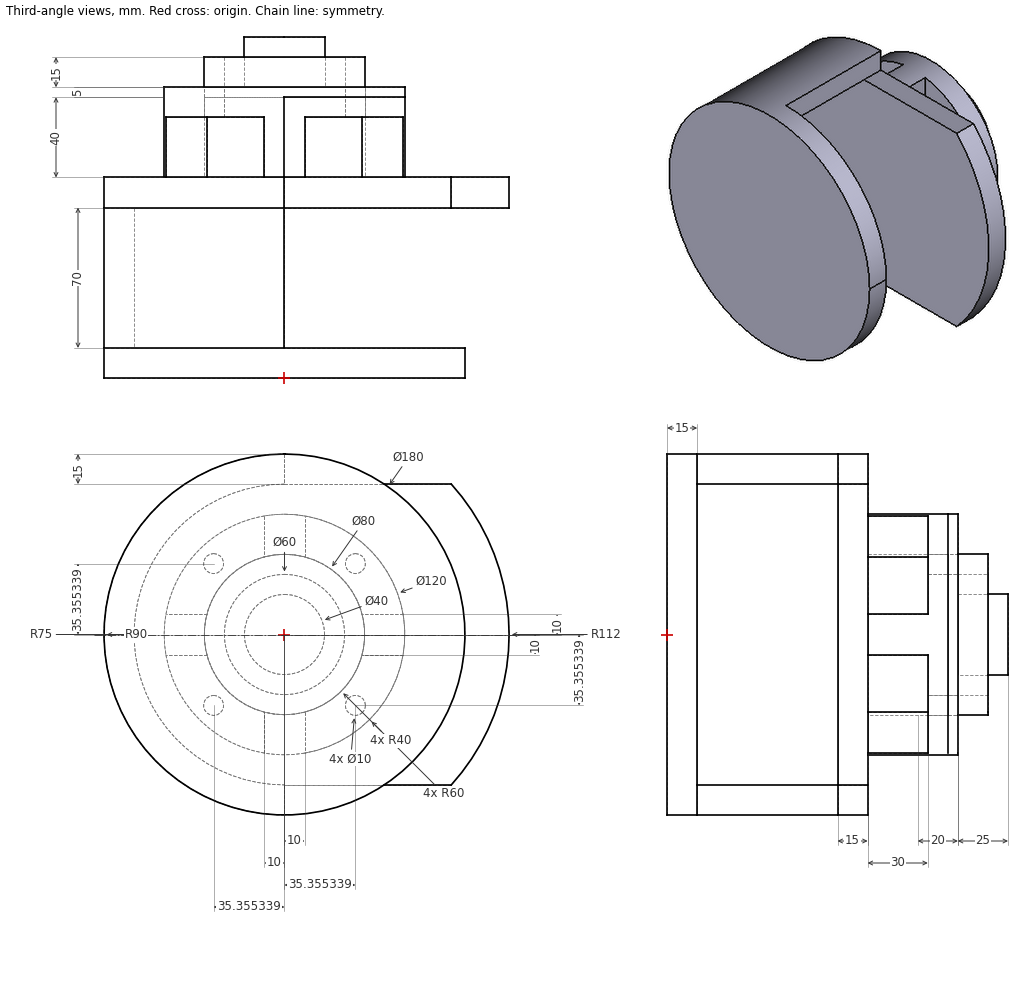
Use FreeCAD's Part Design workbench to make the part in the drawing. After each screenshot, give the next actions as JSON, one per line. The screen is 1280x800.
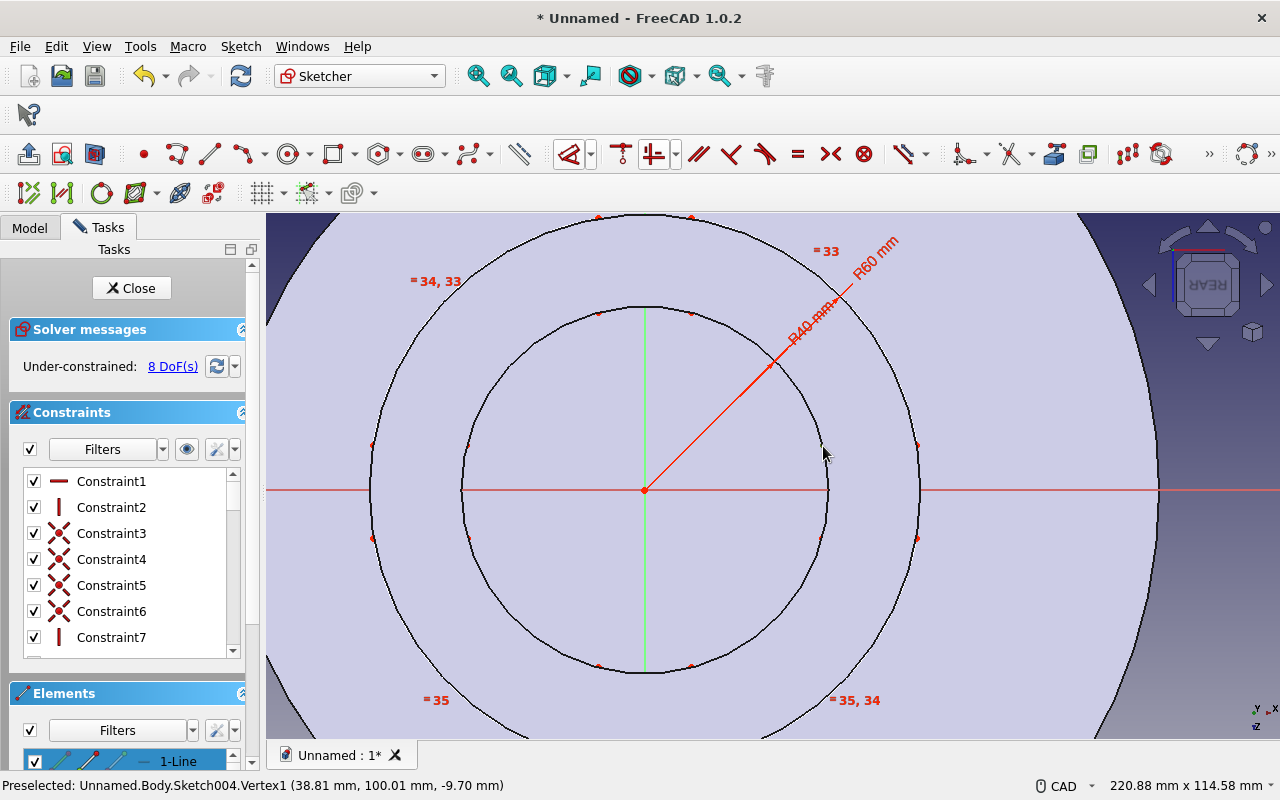
{"action": "left_click", "coordinate": [590, 154]}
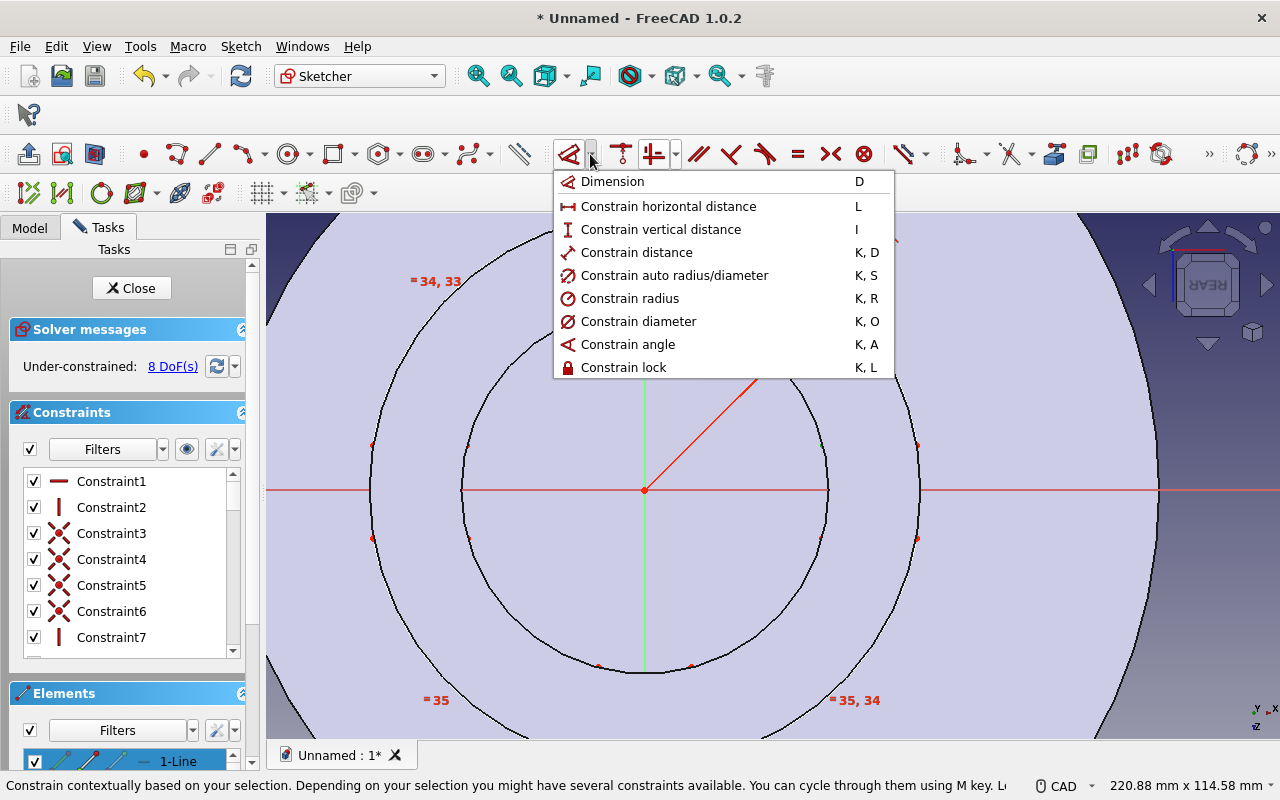
{"action": "left_click", "coordinate": [724, 230]}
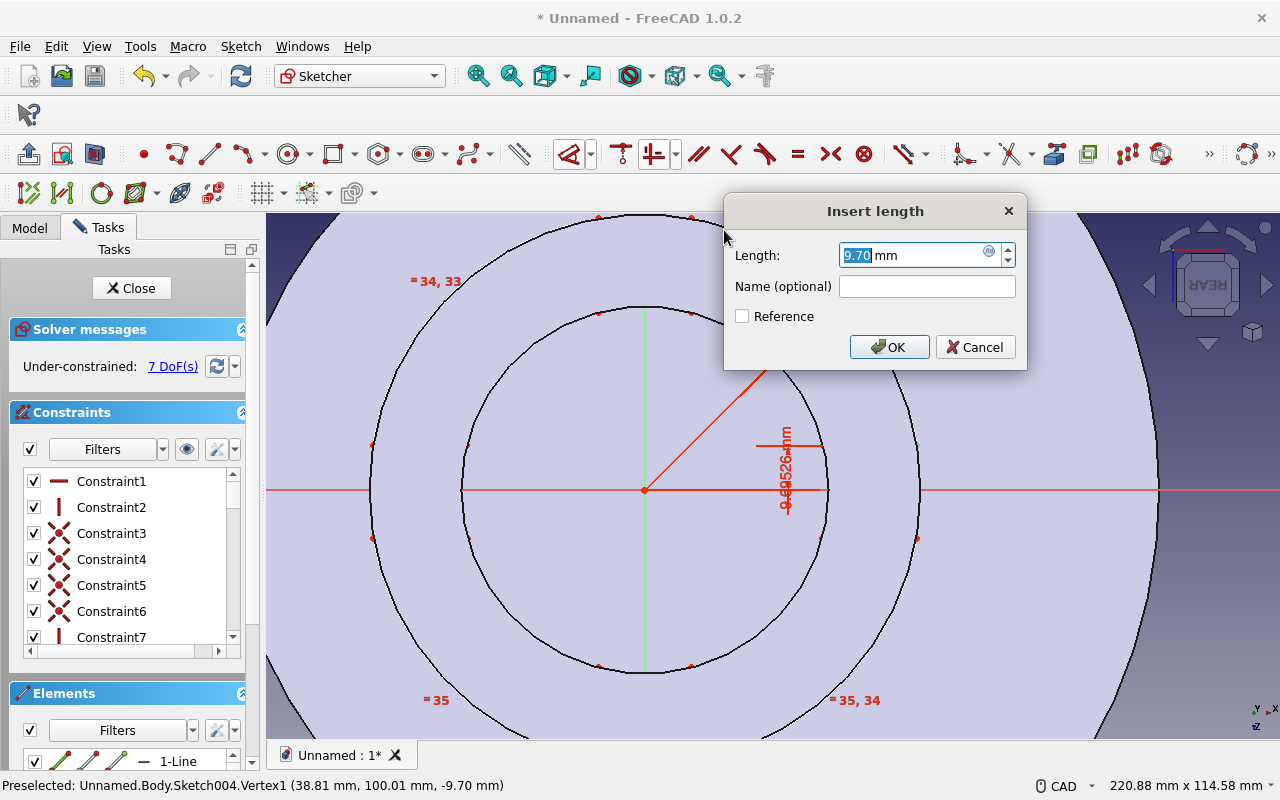
{"action": "type", "text": "10"}
{"action": "key", "text": "Return"}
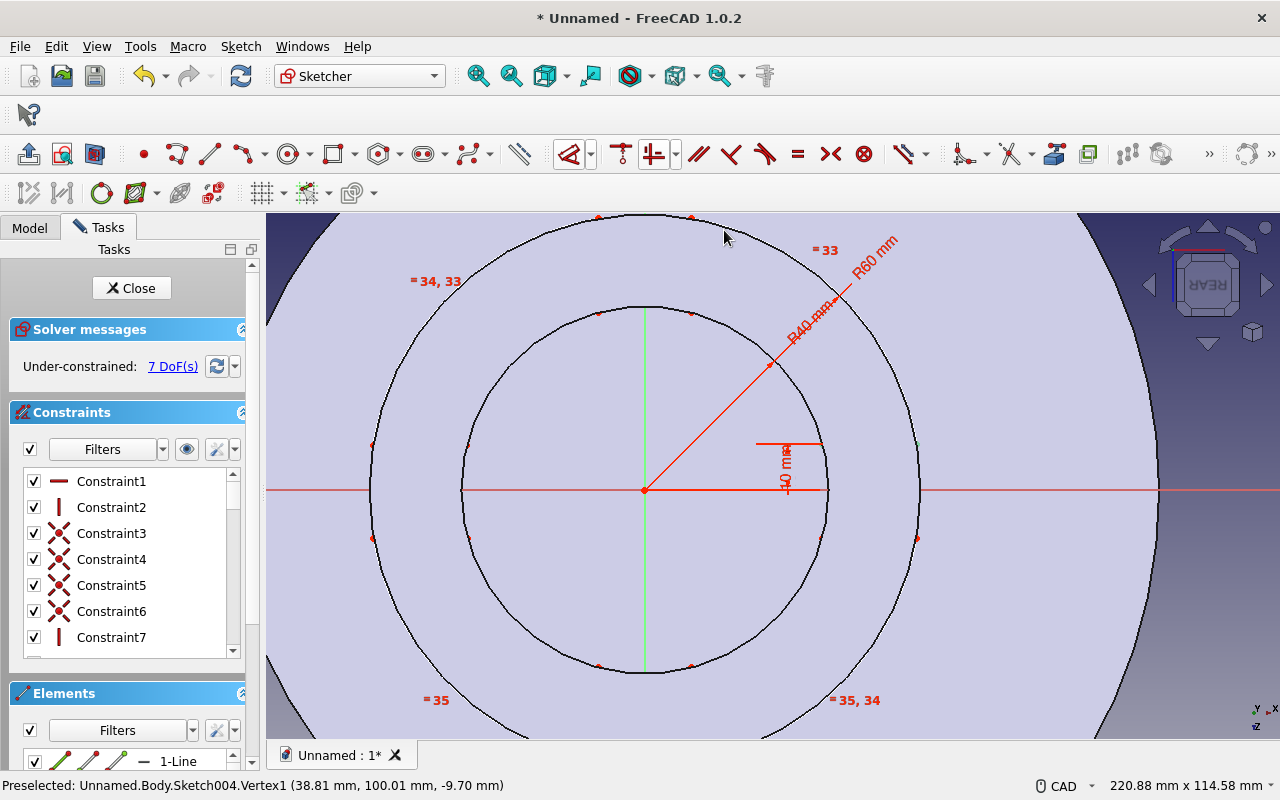
{"action": "scroll", "coordinate": [826, 447], "scroll_direction": "down", "scroll_amount": 2}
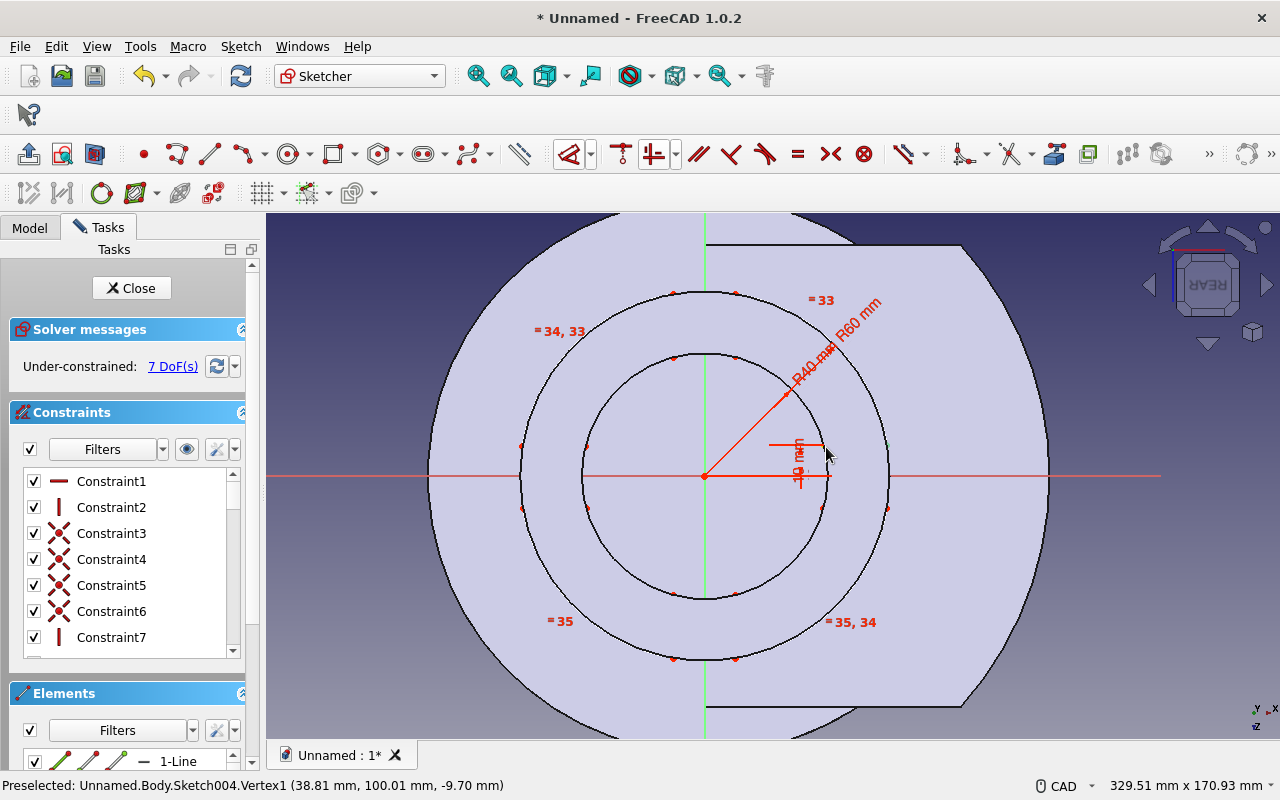
{"action": "scroll", "coordinate": [736, 294], "scroll_direction": "up", "scroll_amount": 2}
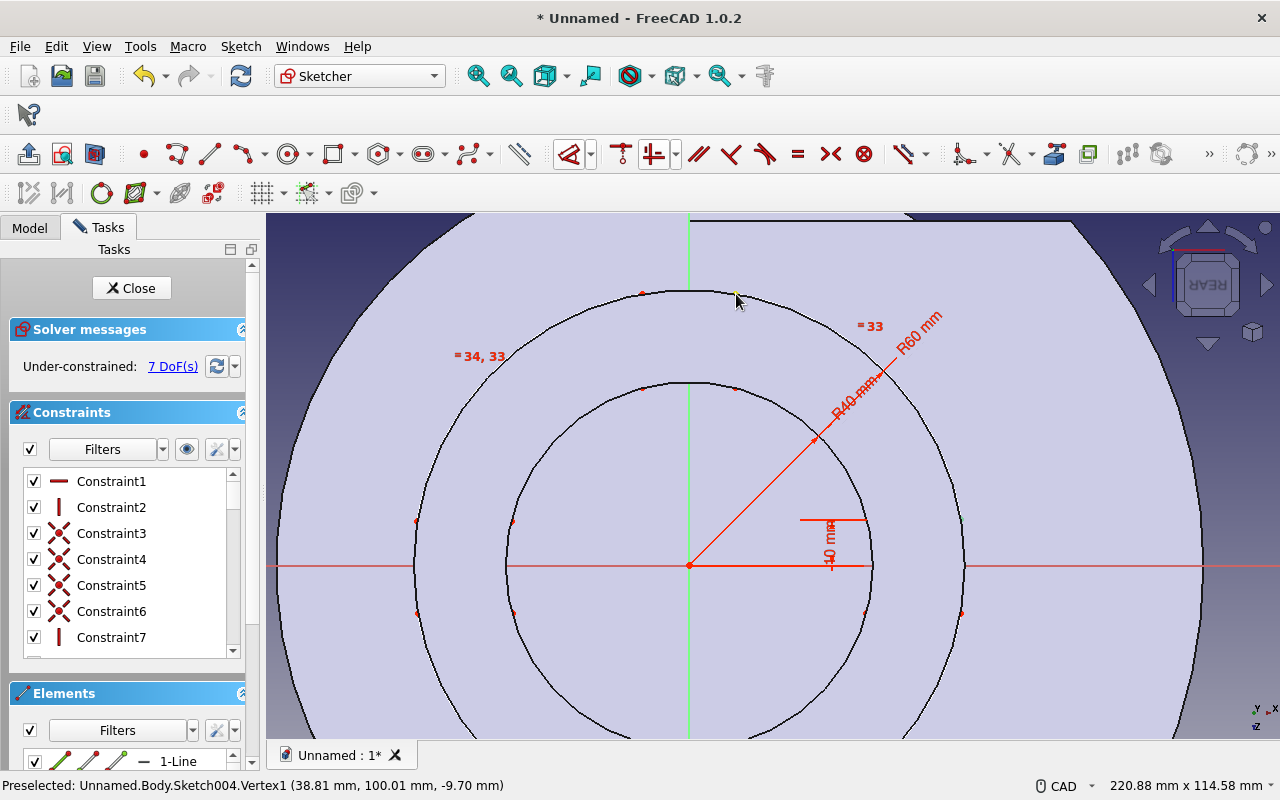
{"action": "left_click", "coordinate": [735, 294]}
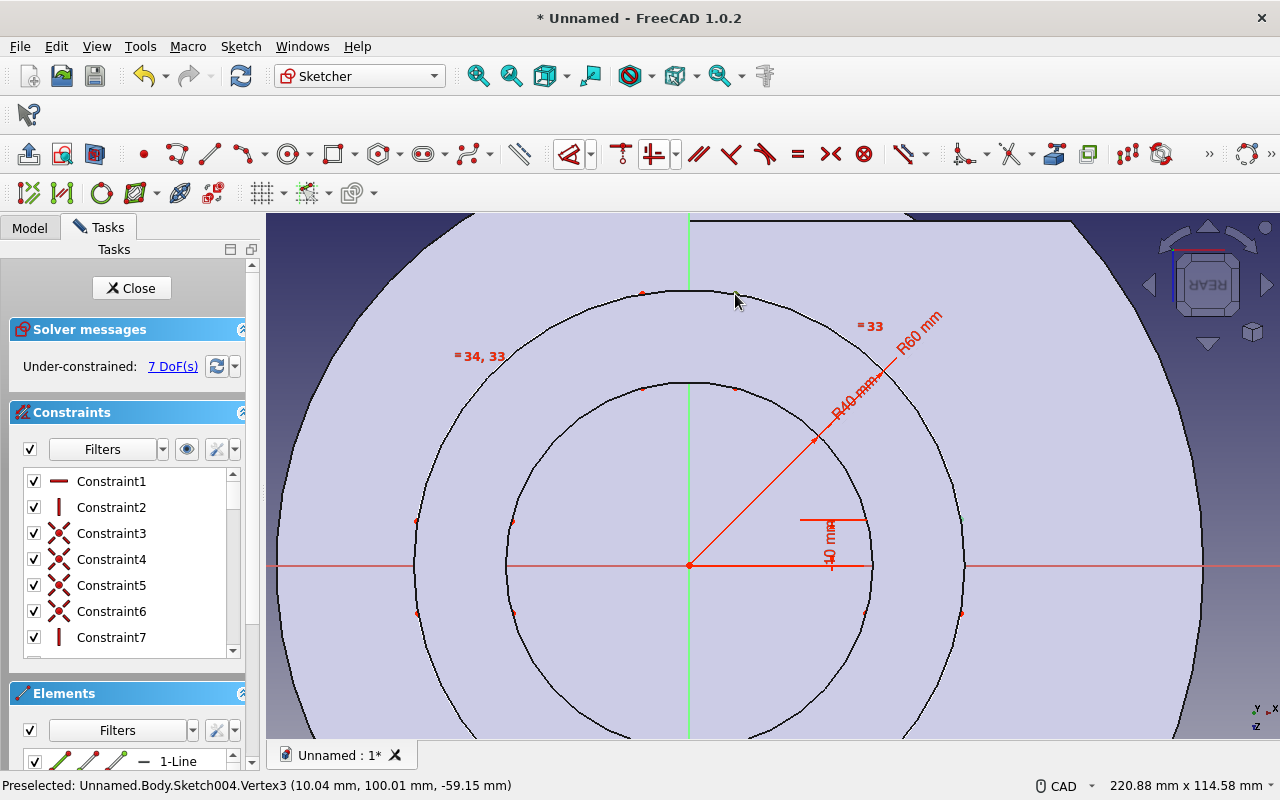
{"action": "left_click", "coordinate": [590, 154]}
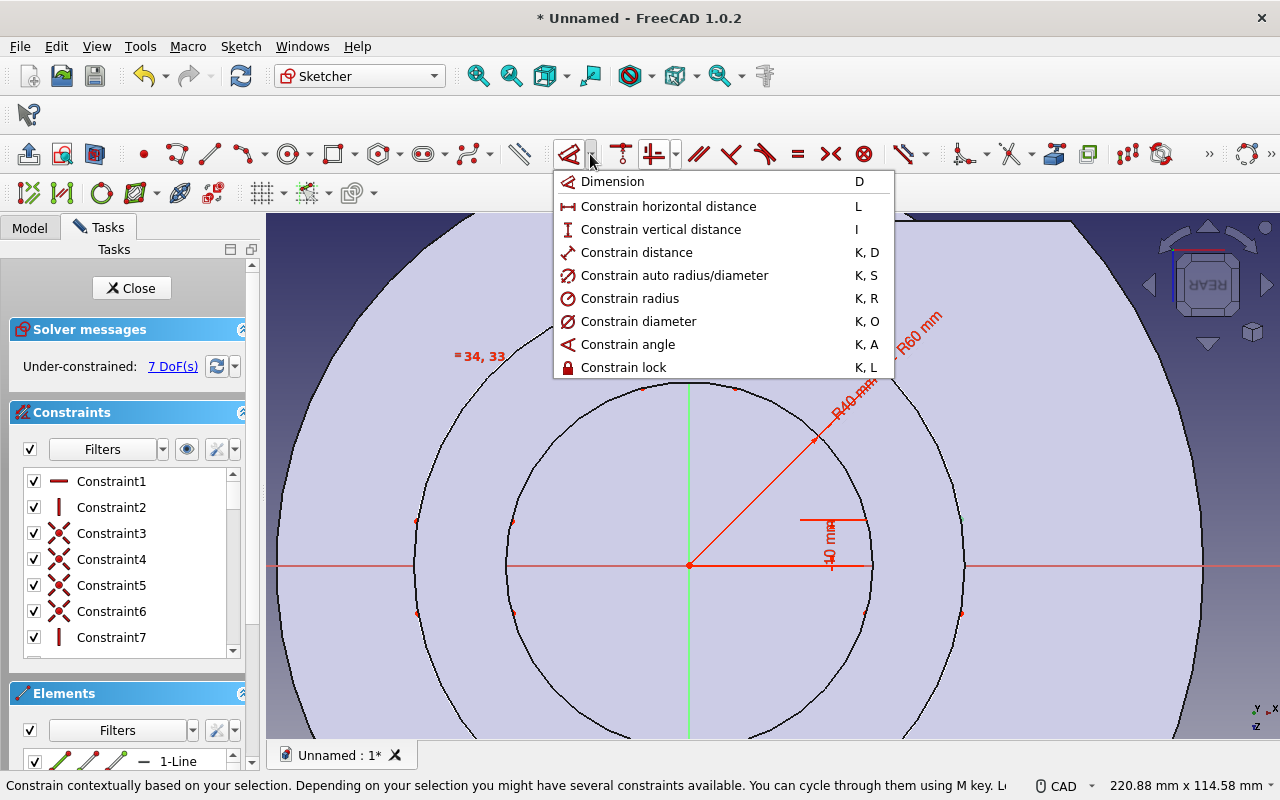
{"action": "left_click", "coordinate": [724, 206]}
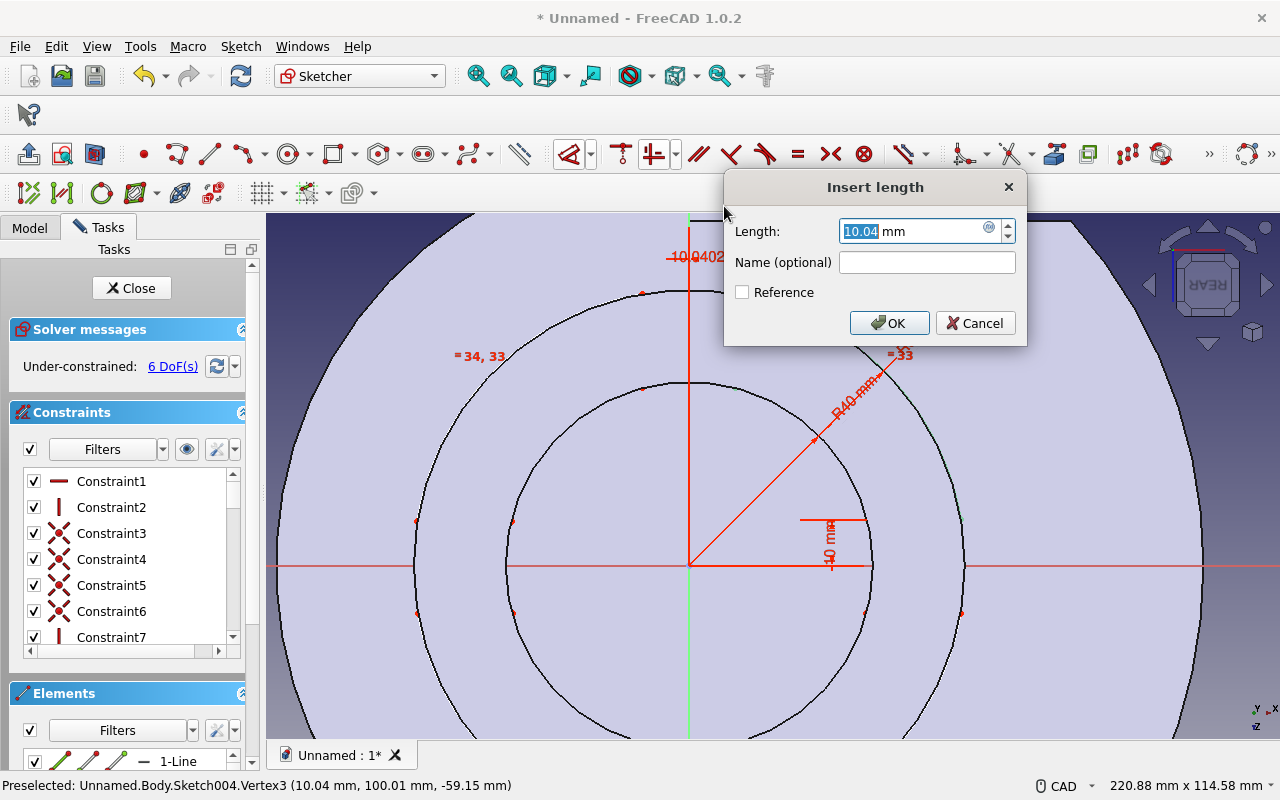
{"action": "type", "text": "10"}
{"action": "key", "text": "Return"}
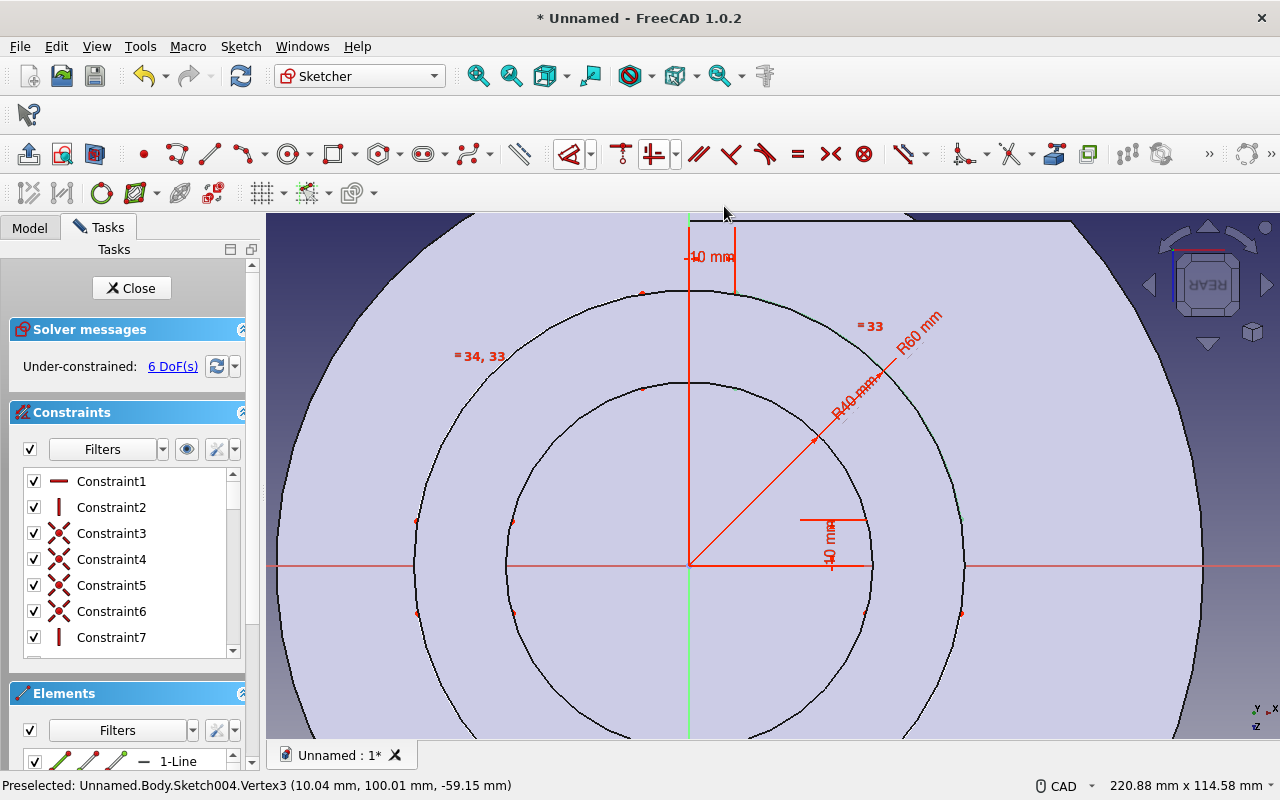
{"action": "left_click", "coordinate": [643, 388]}